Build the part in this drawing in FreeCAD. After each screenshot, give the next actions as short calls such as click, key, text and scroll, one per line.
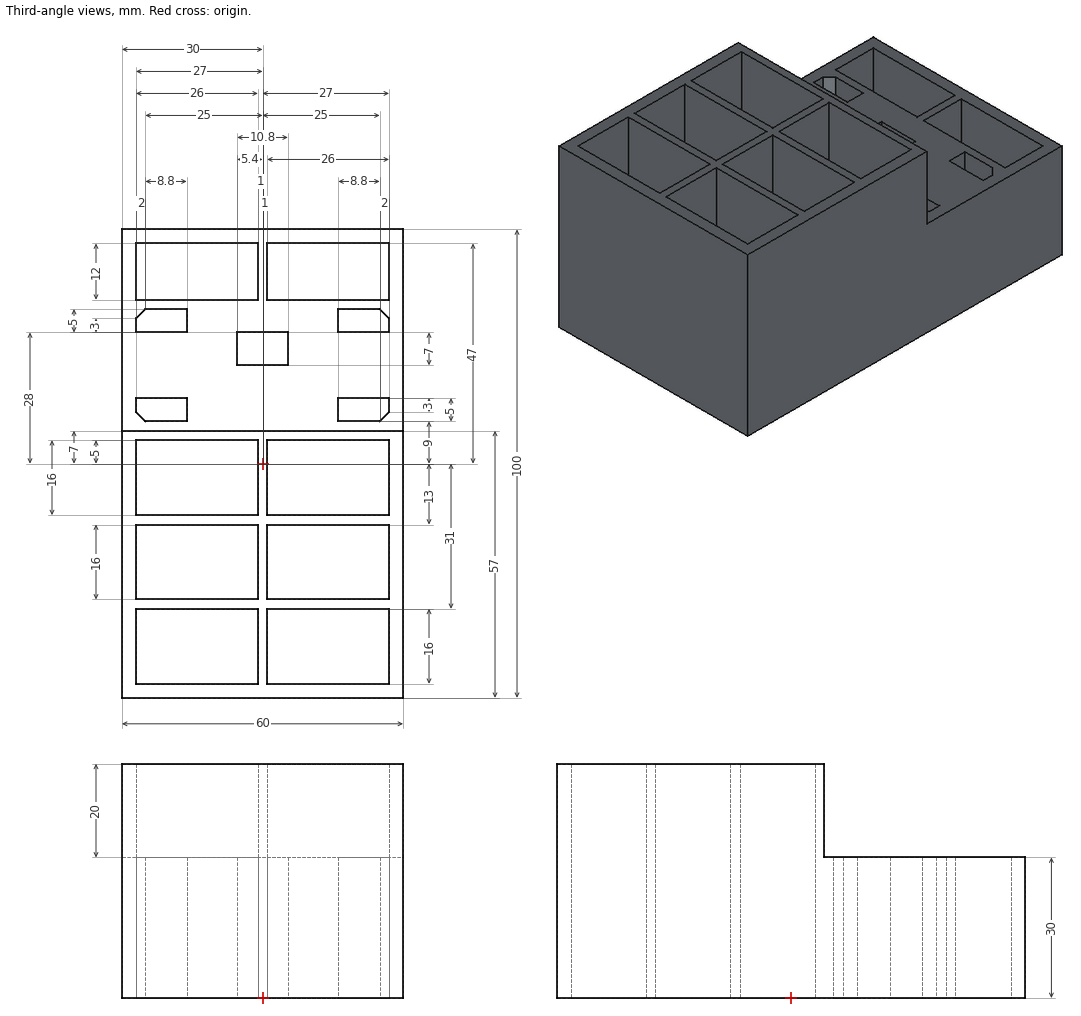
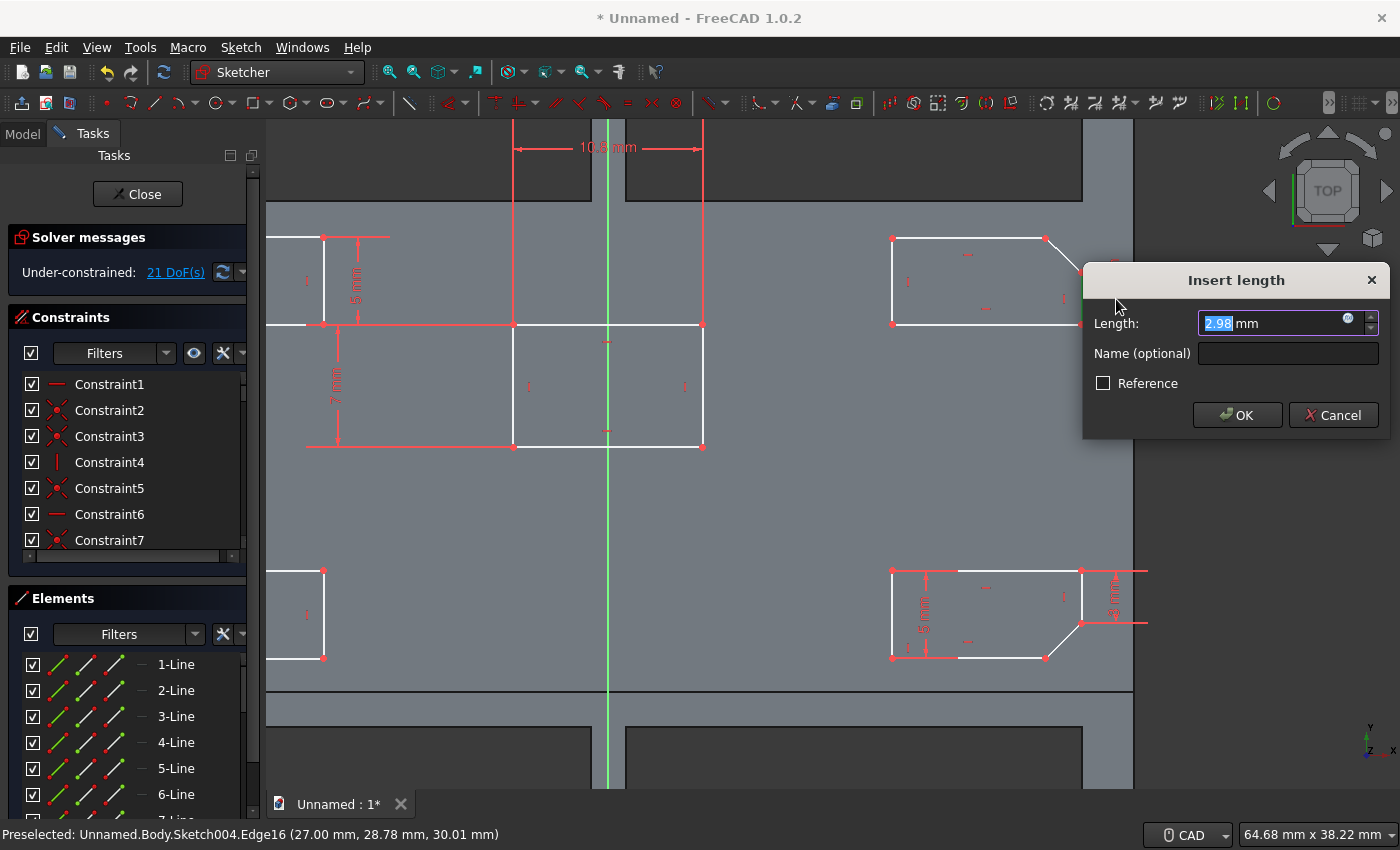
text(3)
key(Return)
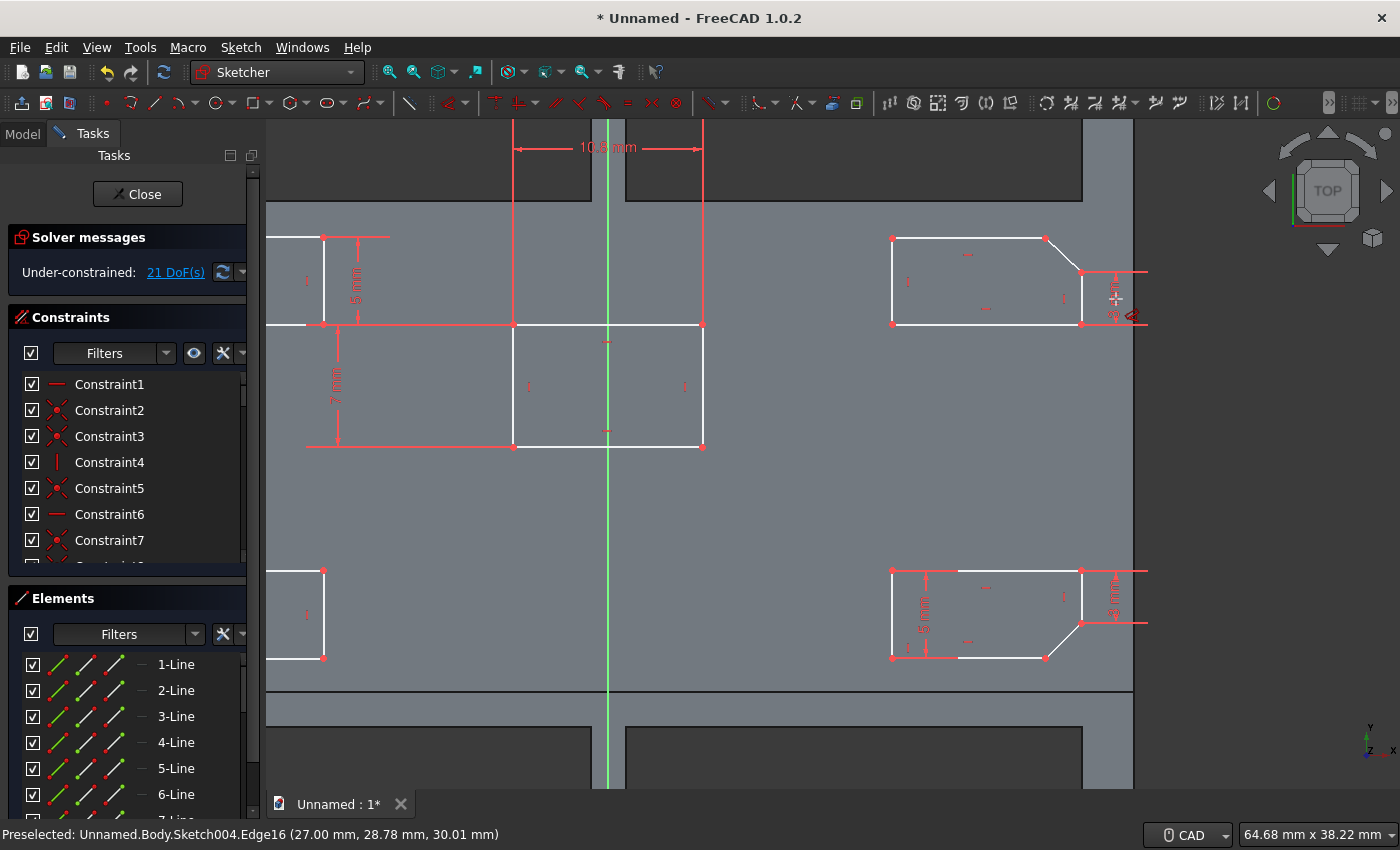
click(892, 264)
click(926, 282)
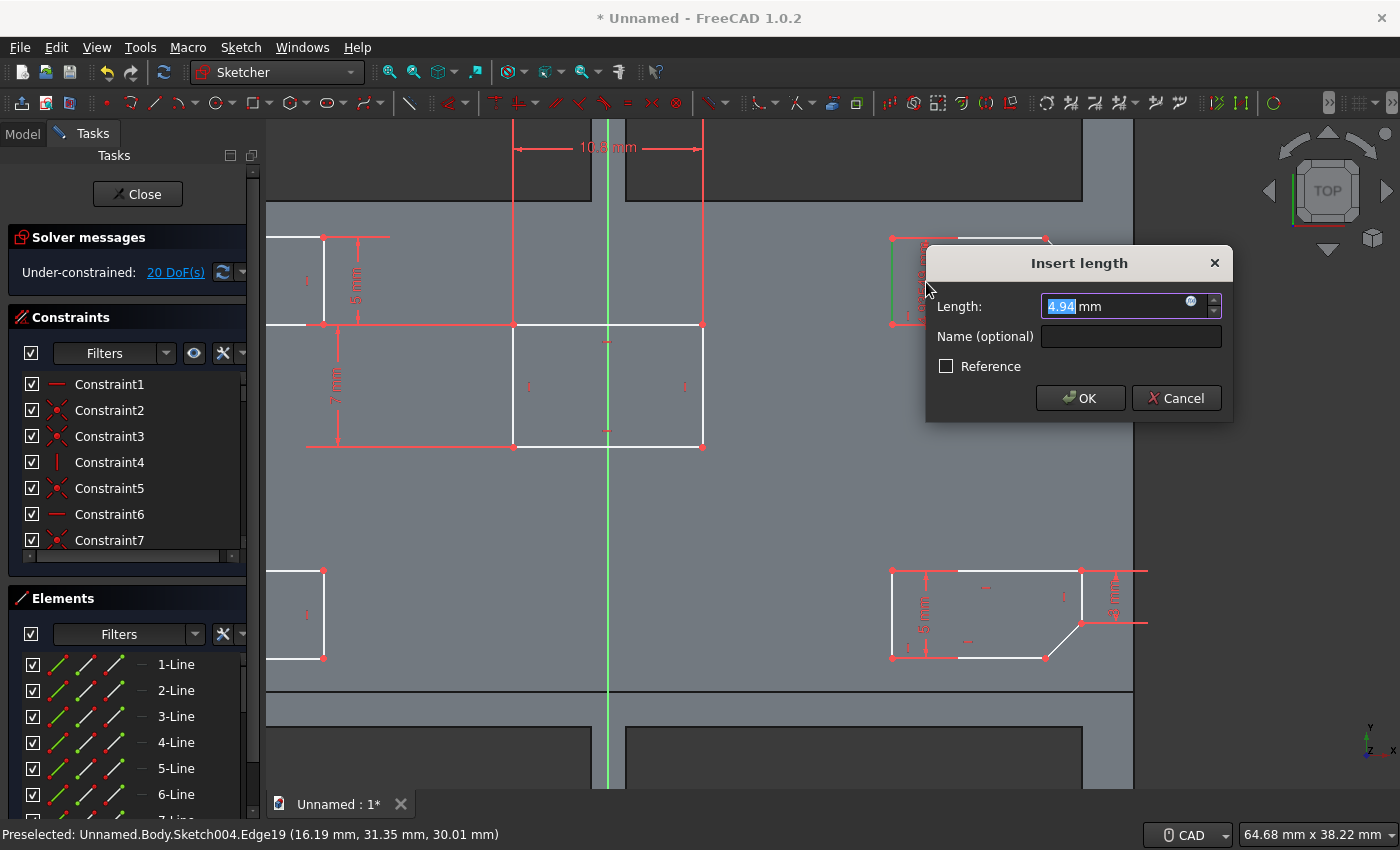
text(5)
key(Return)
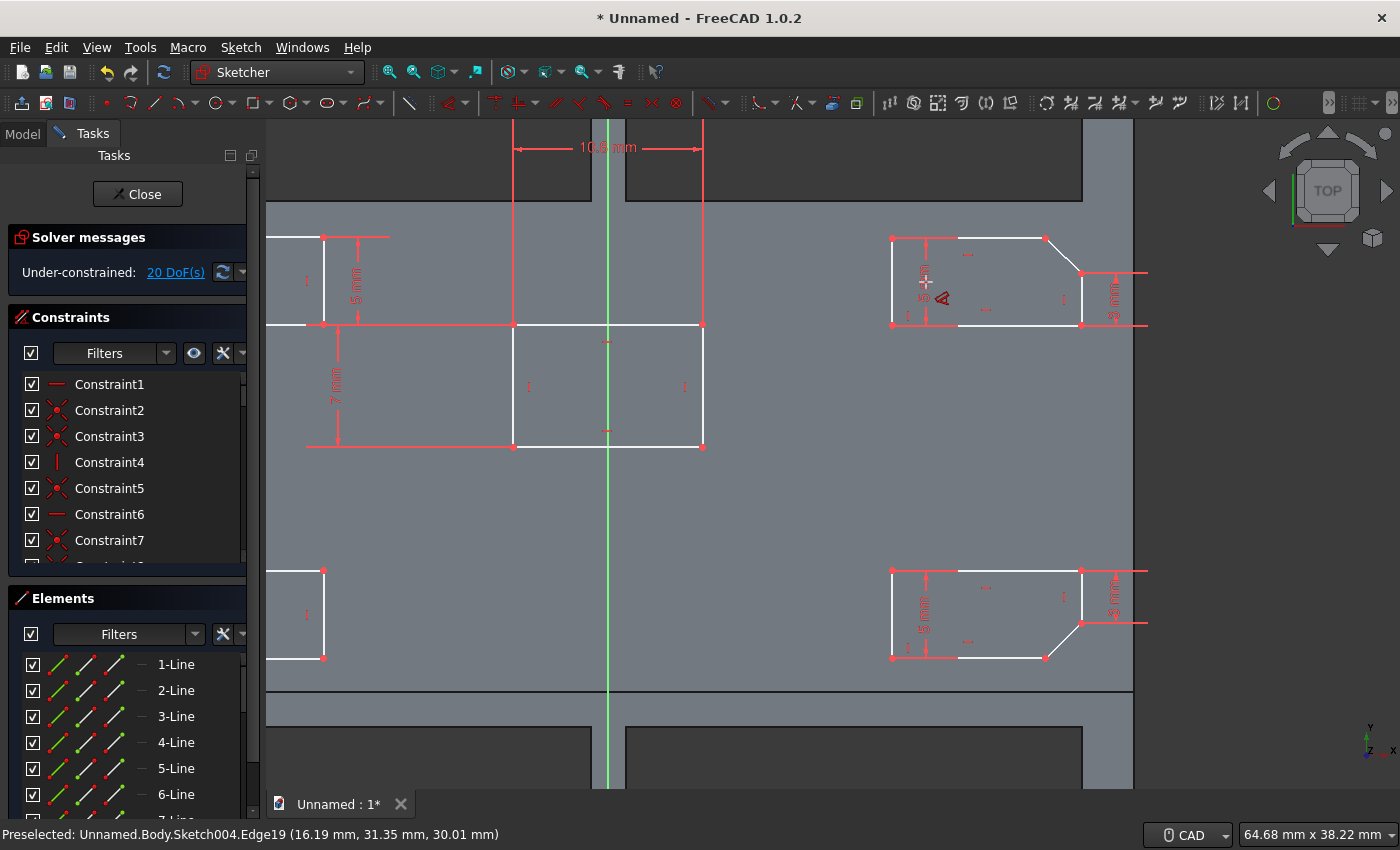
click(324, 633)
click(358, 615)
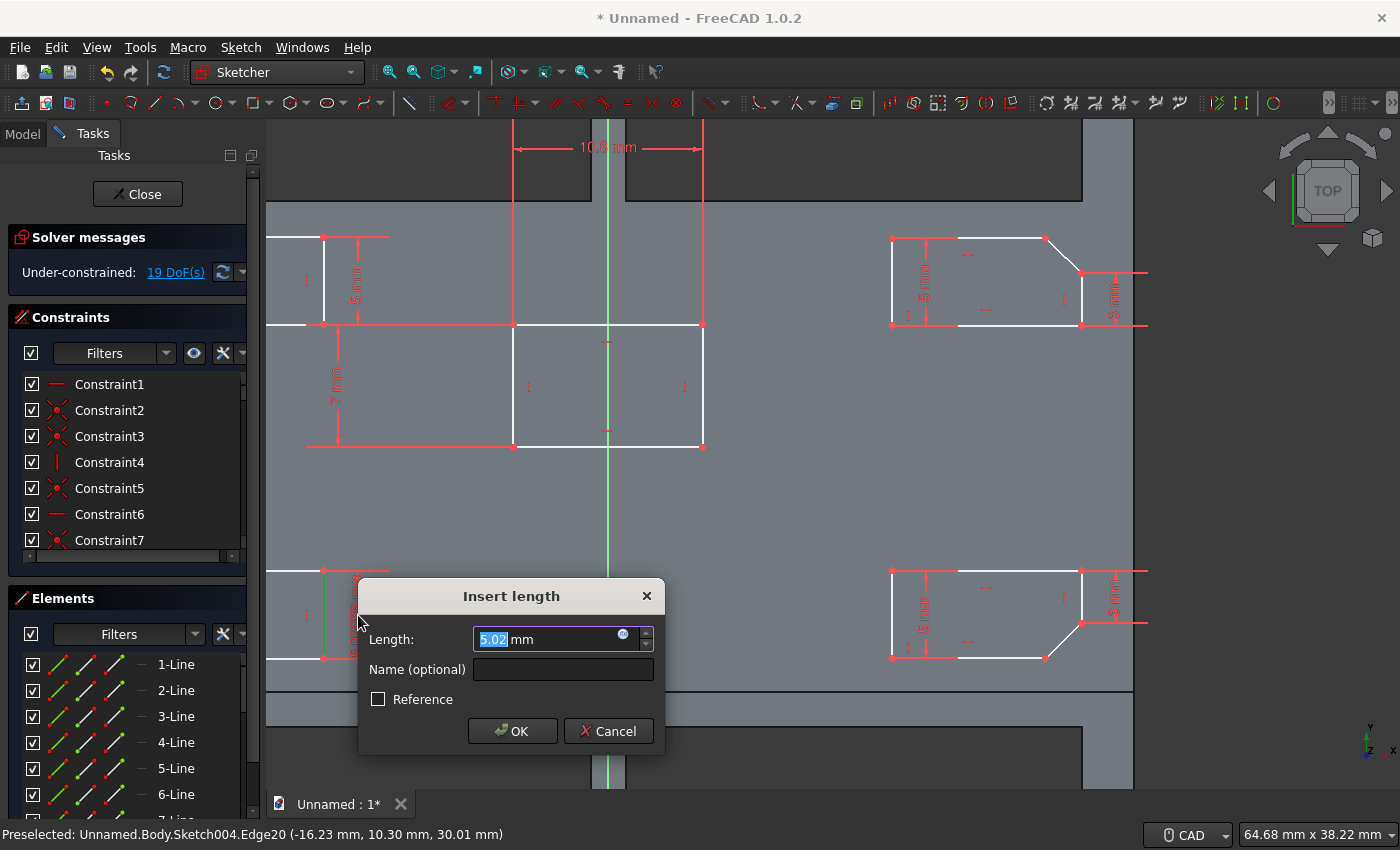
text(5)
key(Return)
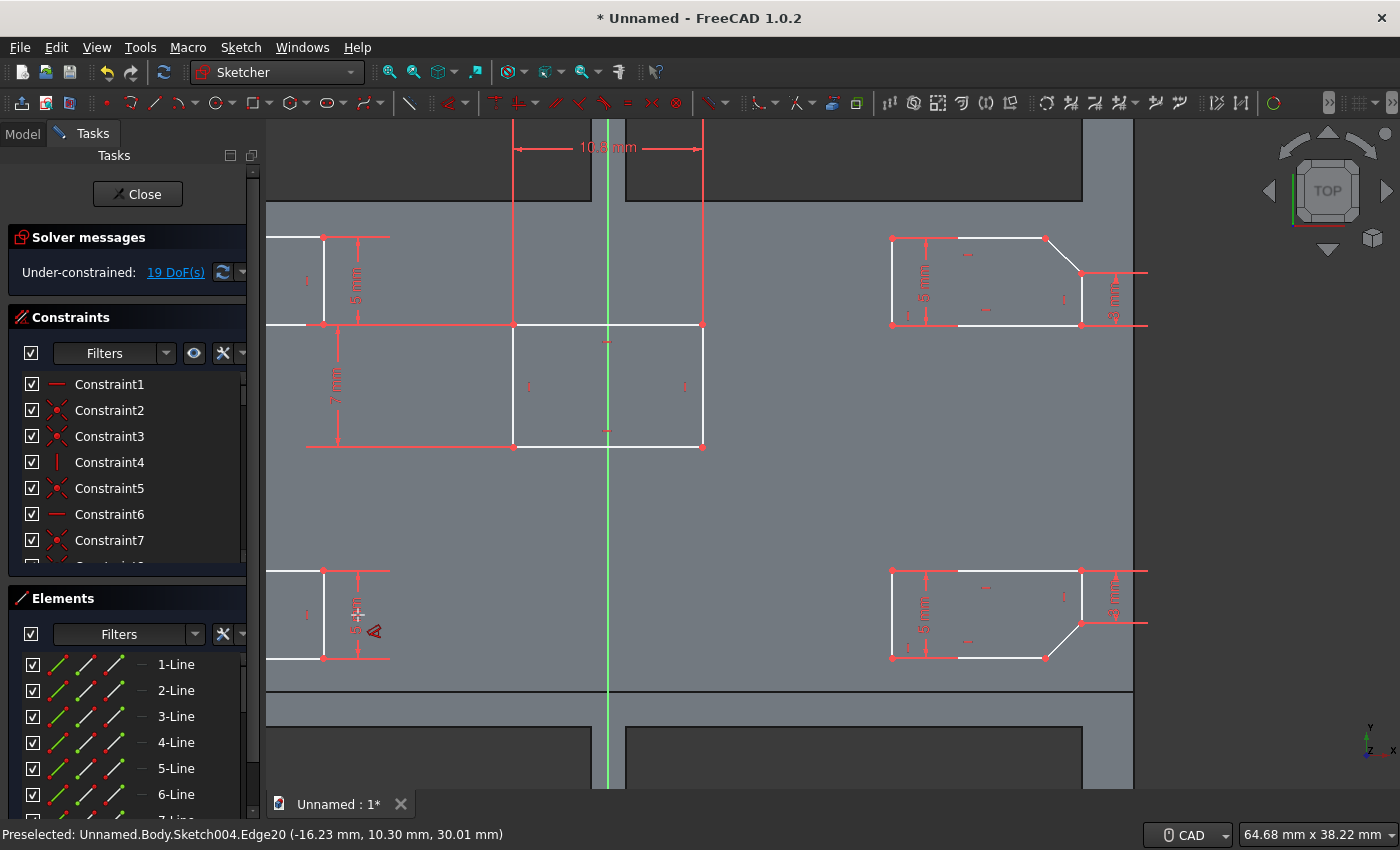
scroll(1082, 309, down, 2)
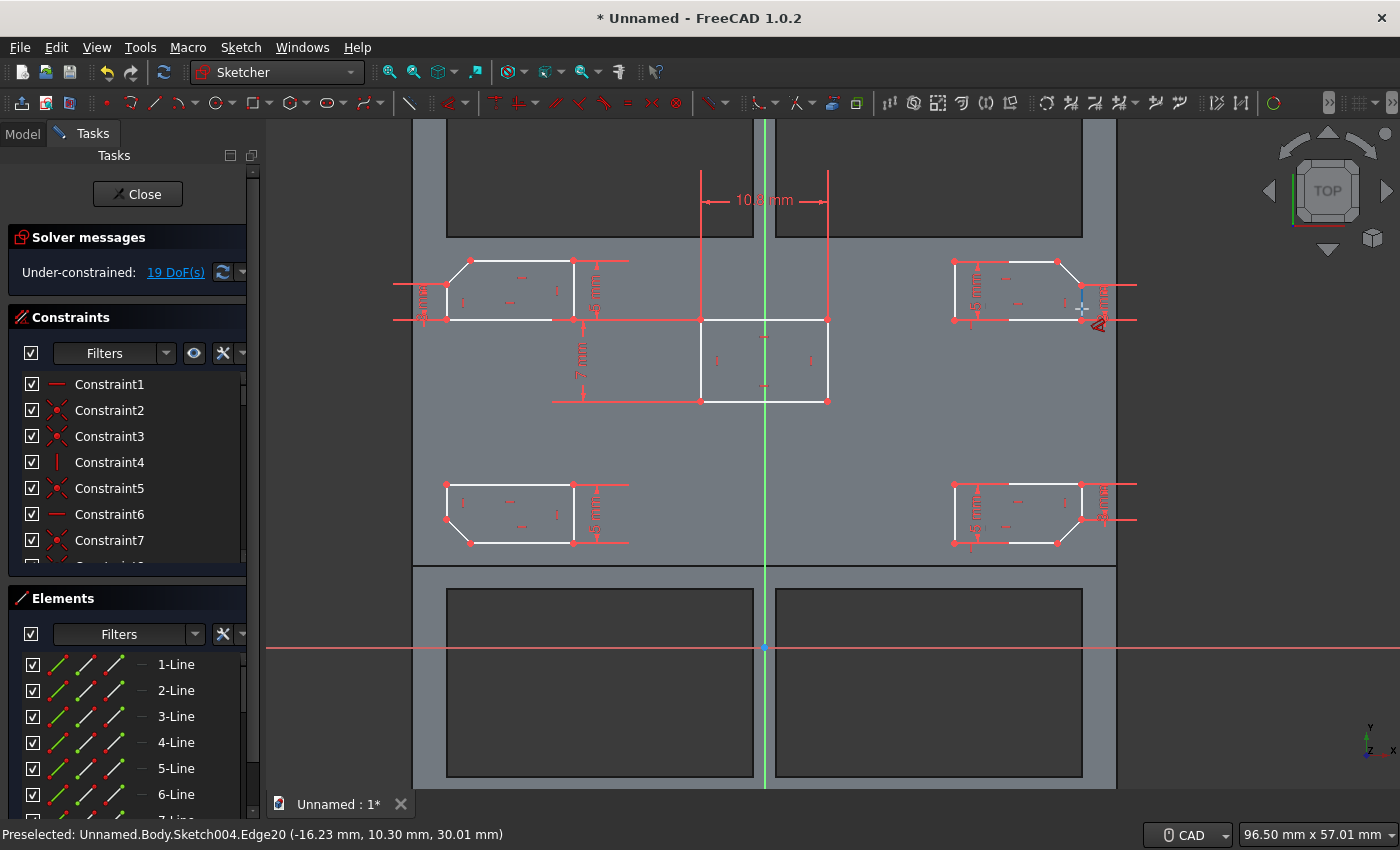
scroll(447, 495, up, 2)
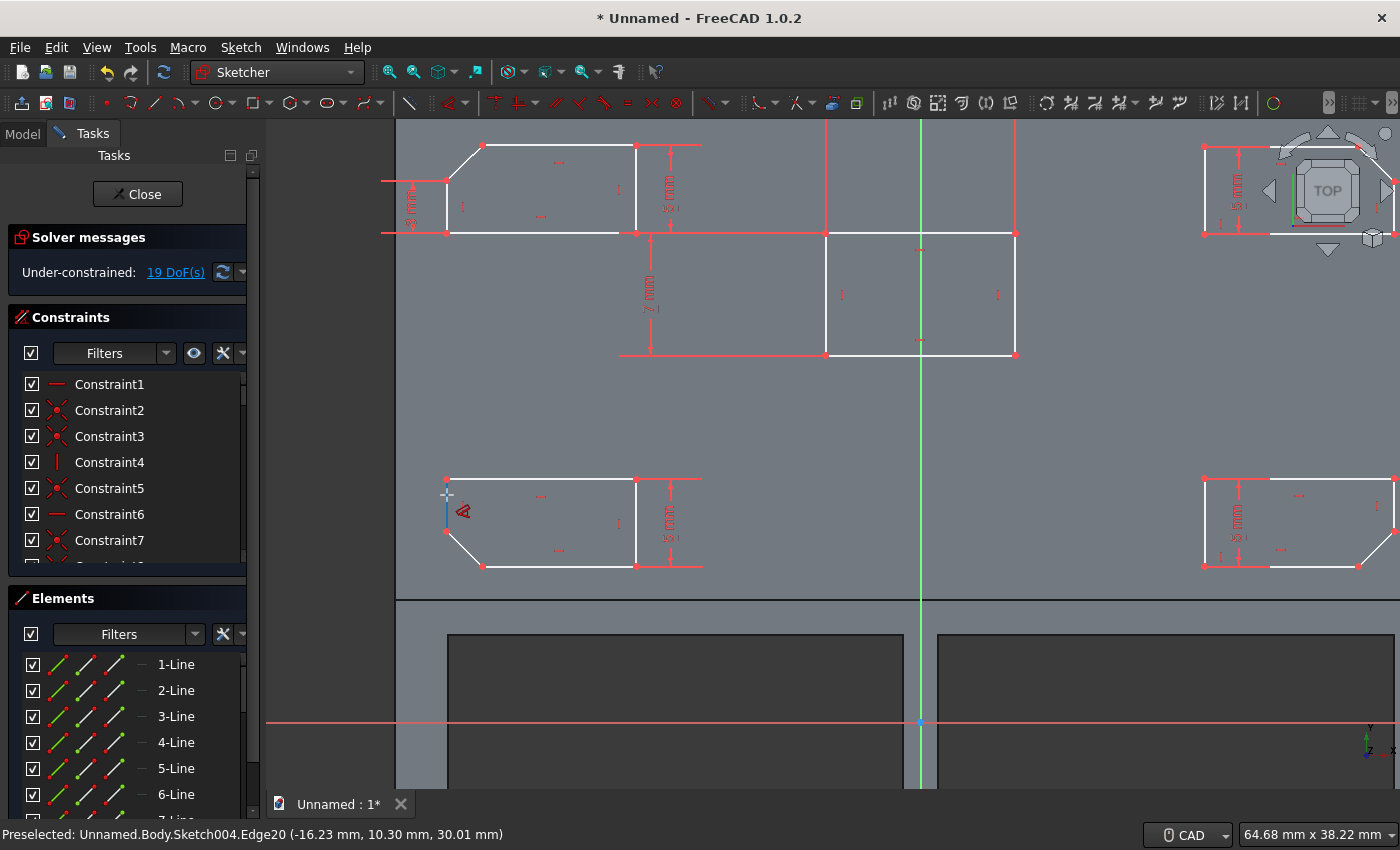
click(447, 495)
click(413, 505)